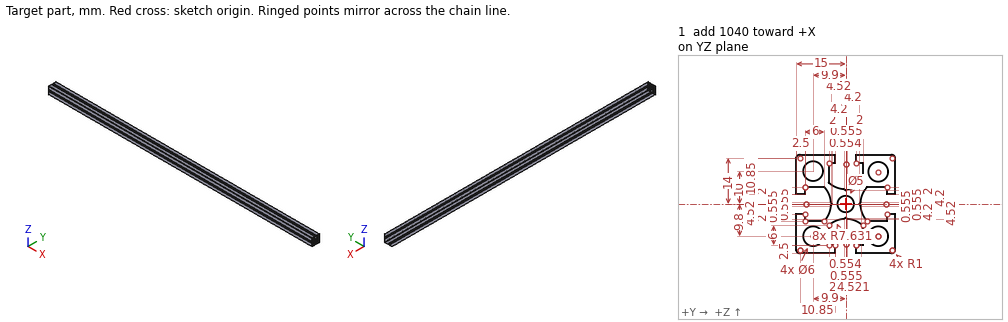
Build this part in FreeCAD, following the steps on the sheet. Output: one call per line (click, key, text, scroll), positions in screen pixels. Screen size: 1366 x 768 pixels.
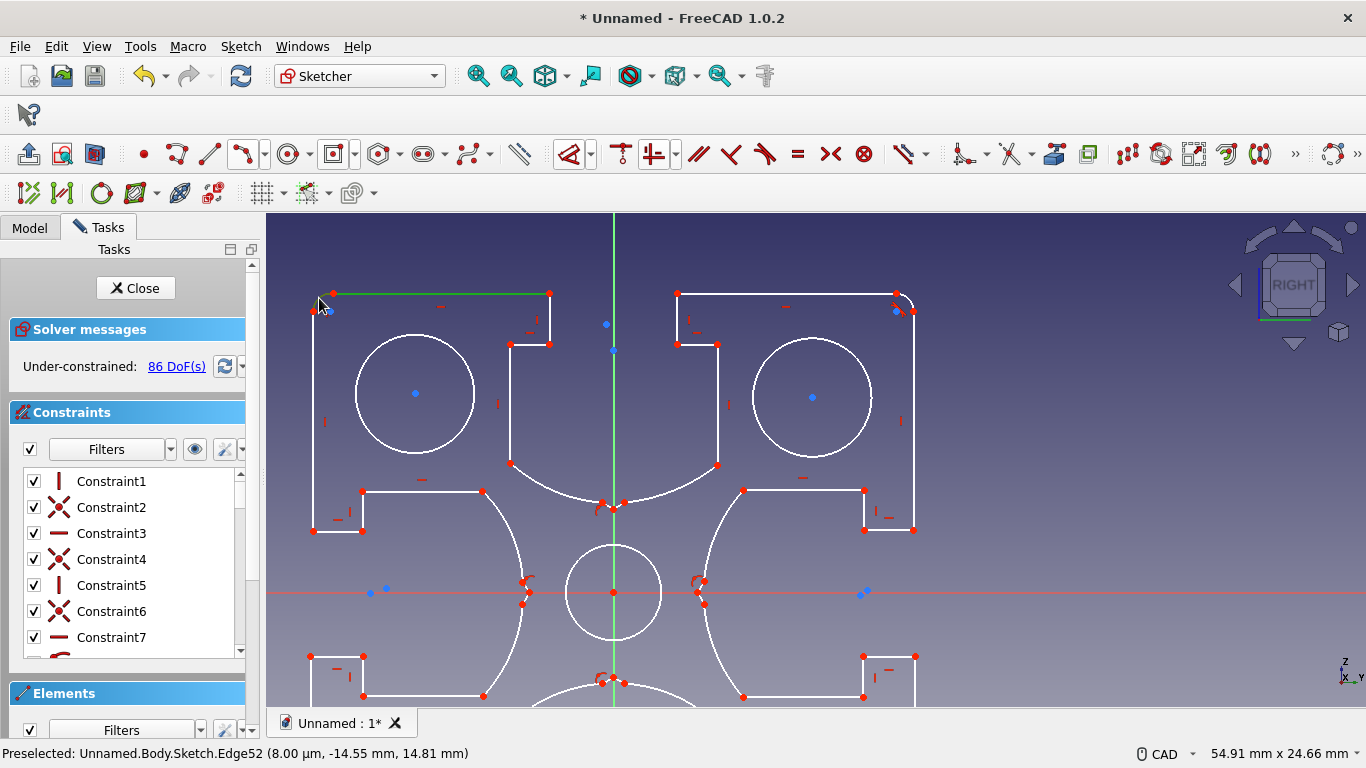
key(t)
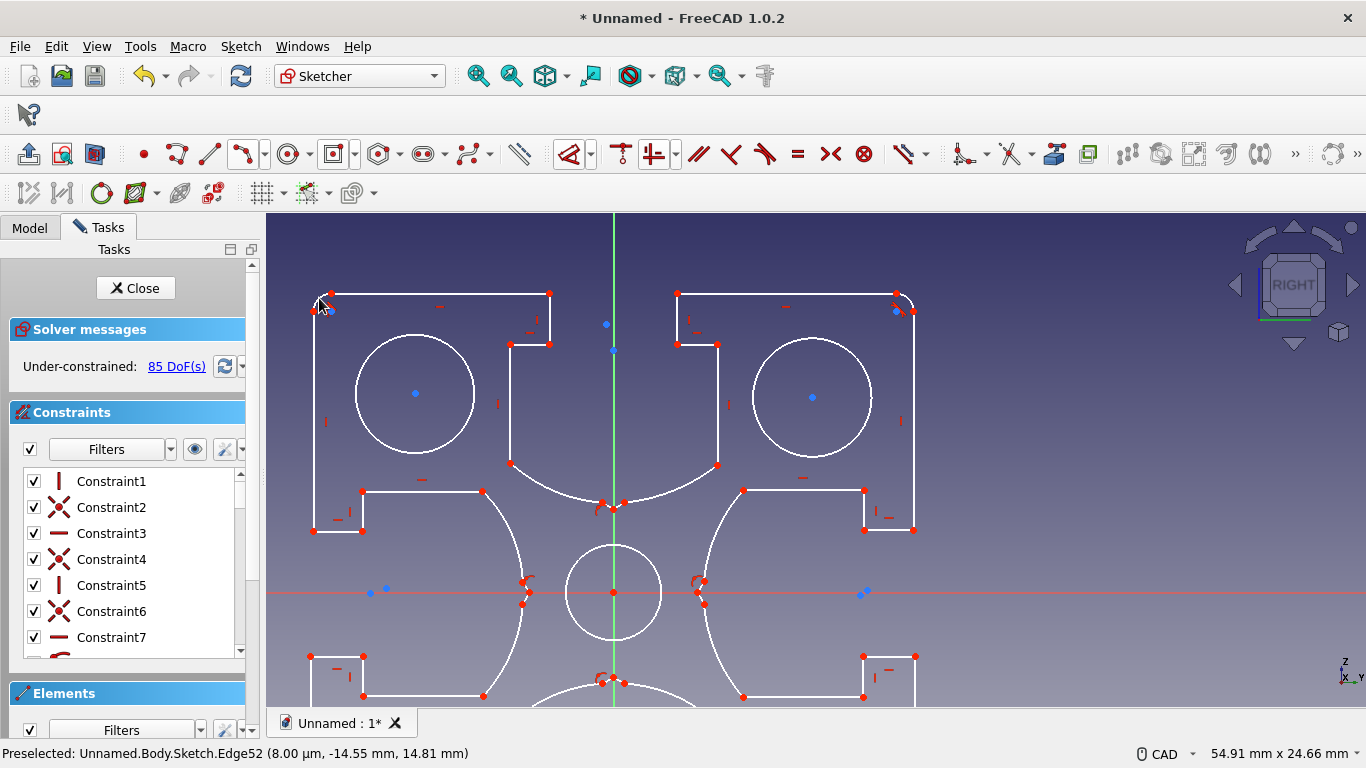
click(518, 552)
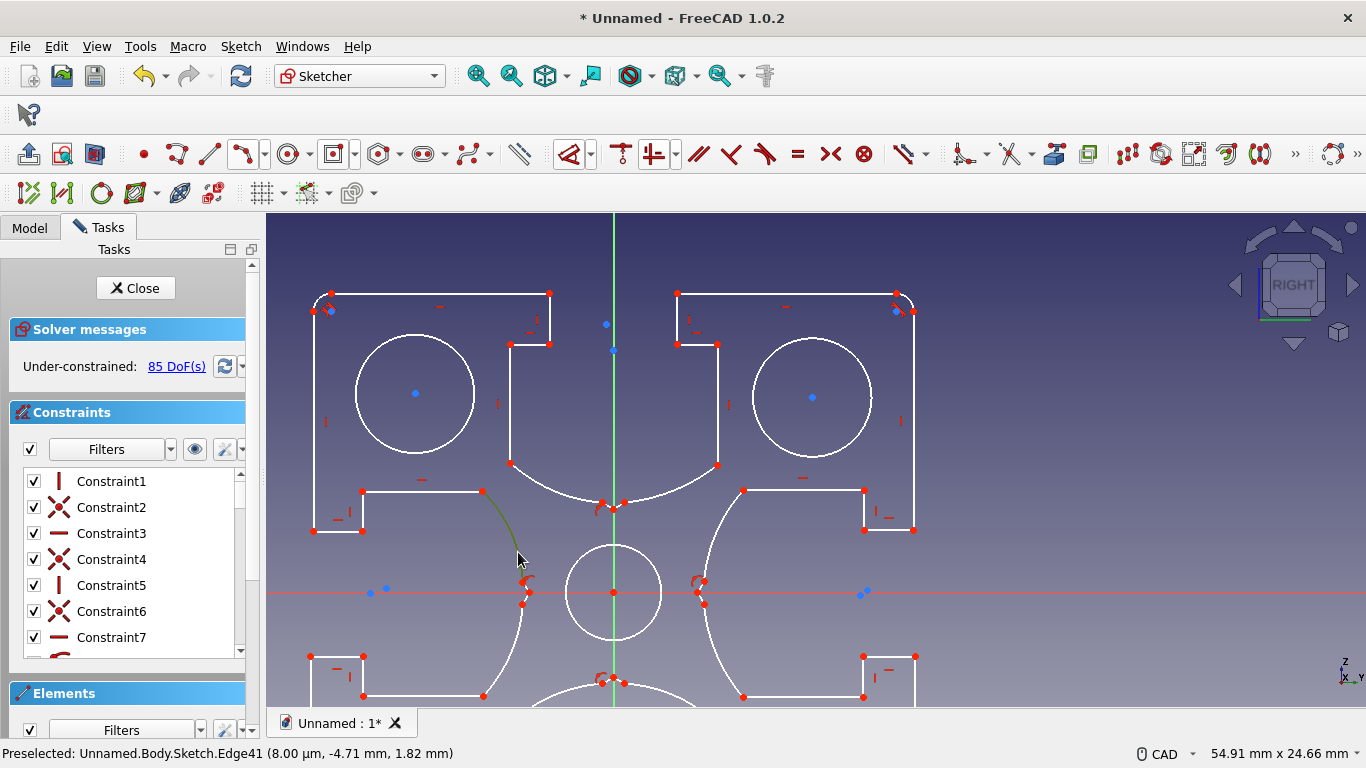
click(502, 672)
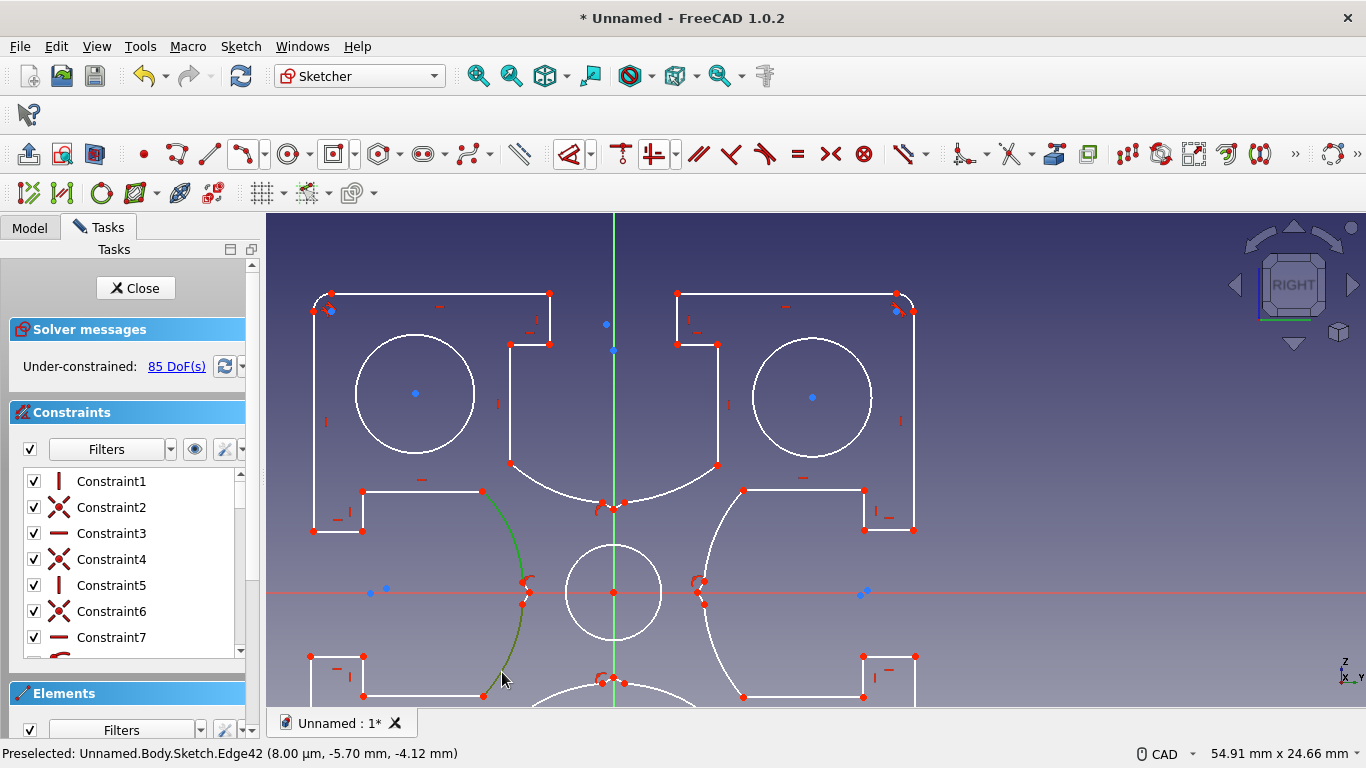
scroll(910, 299, down, 3)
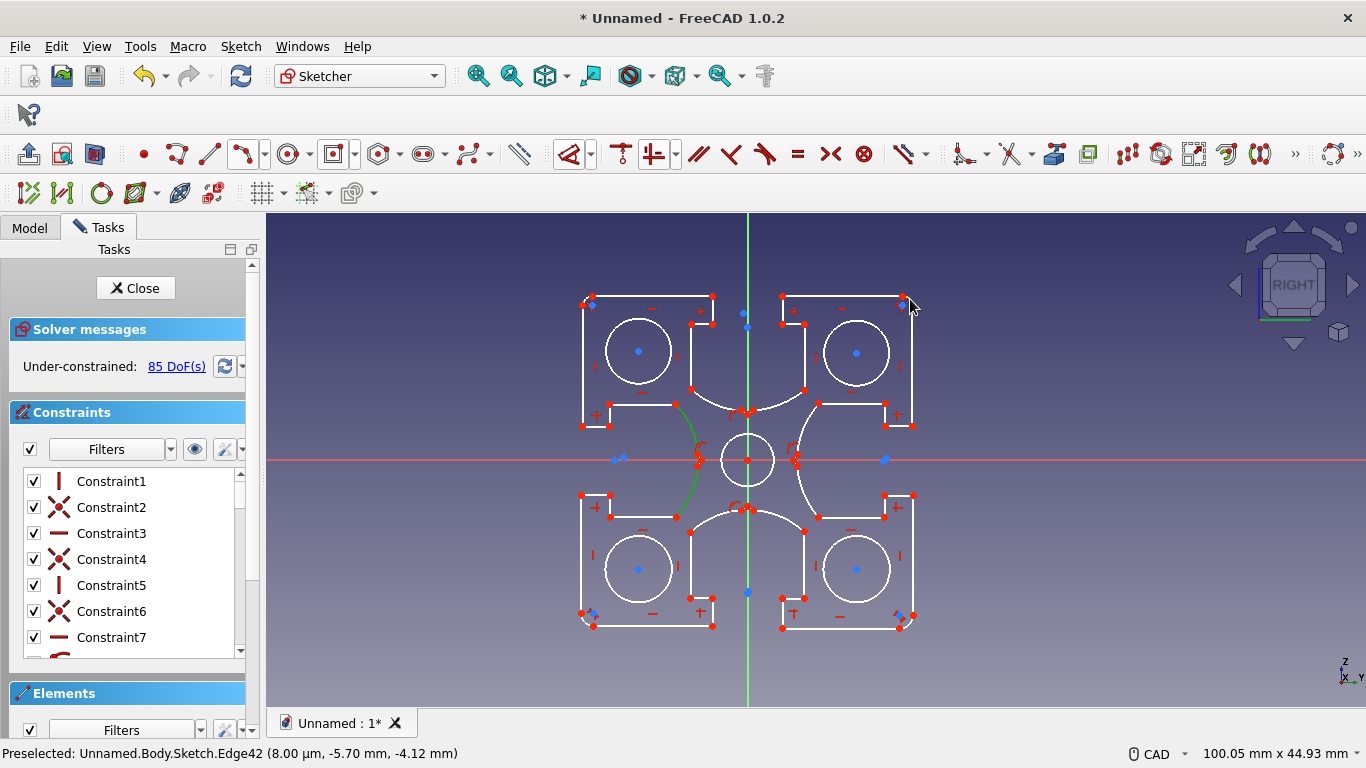
click(725, 513)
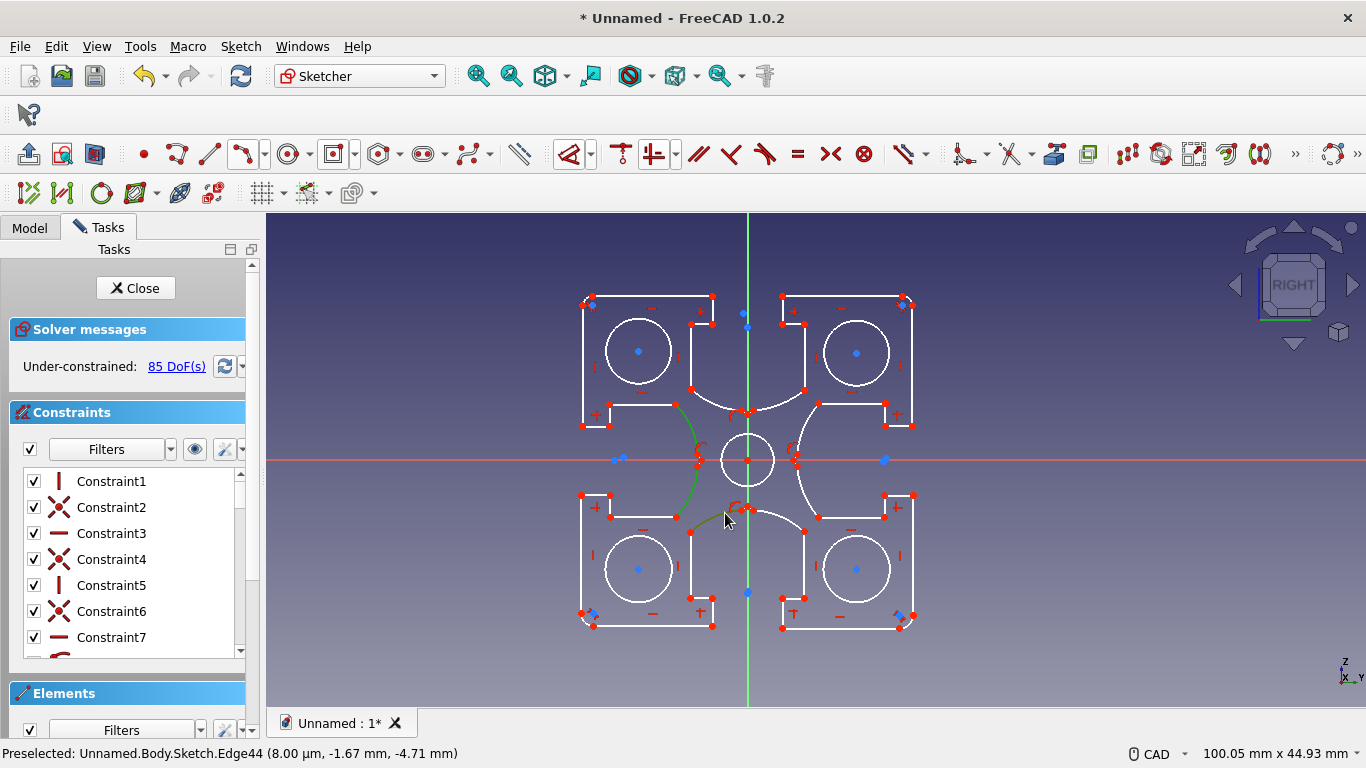
click(791, 522)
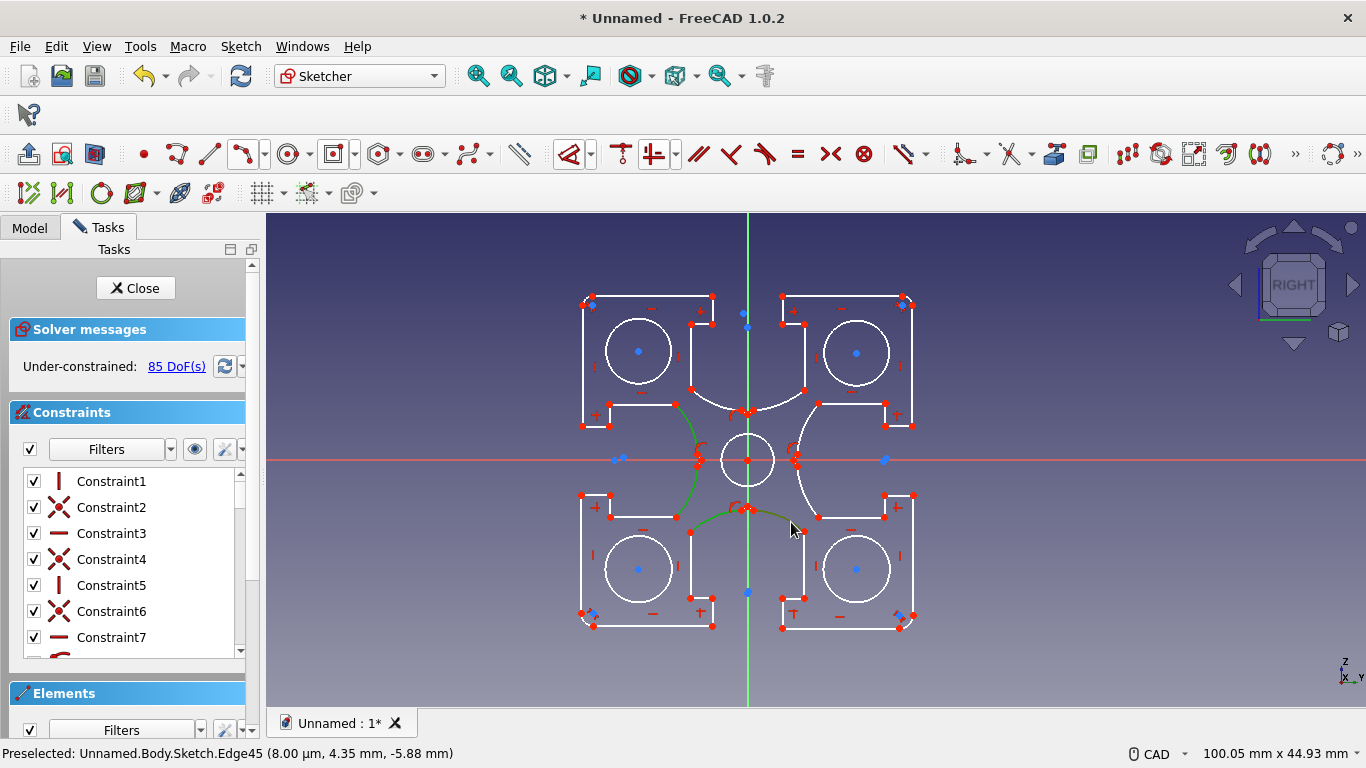
click(800, 483)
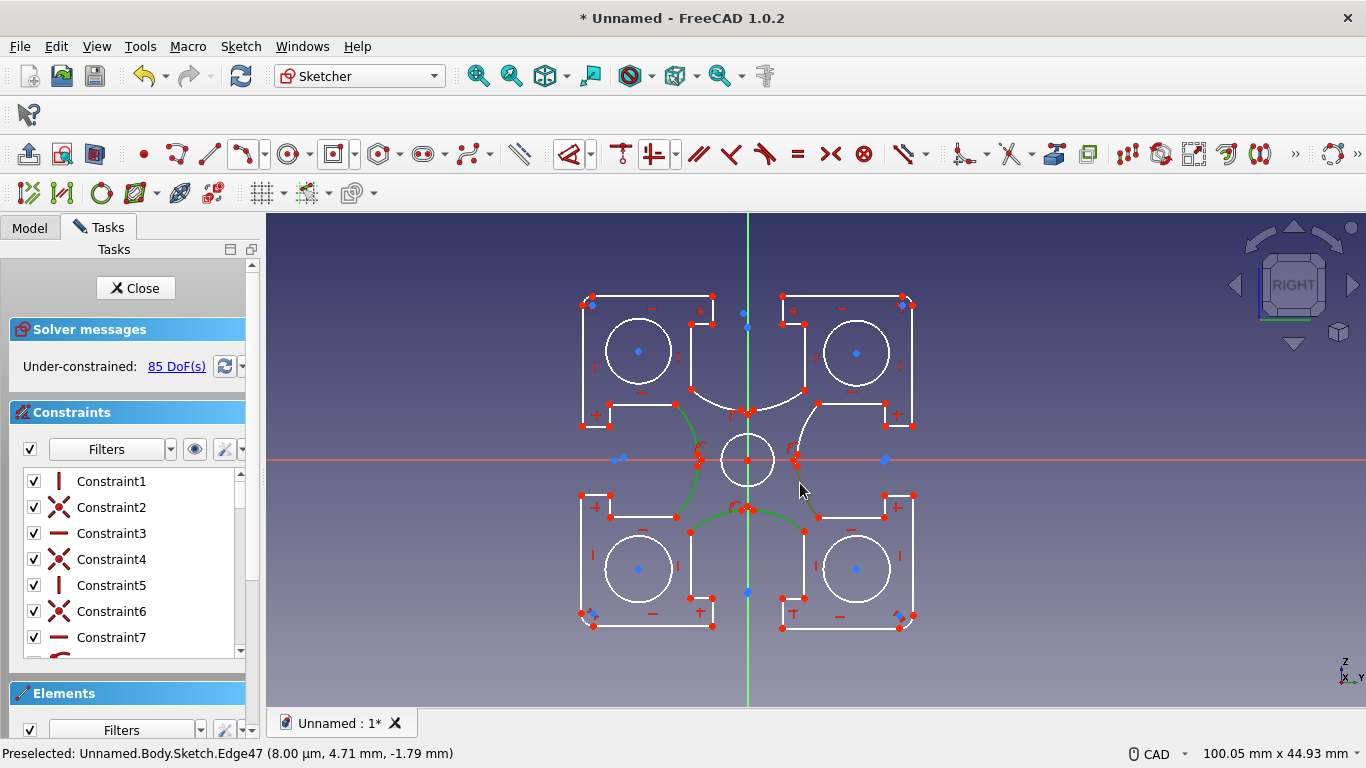
click(809, 417)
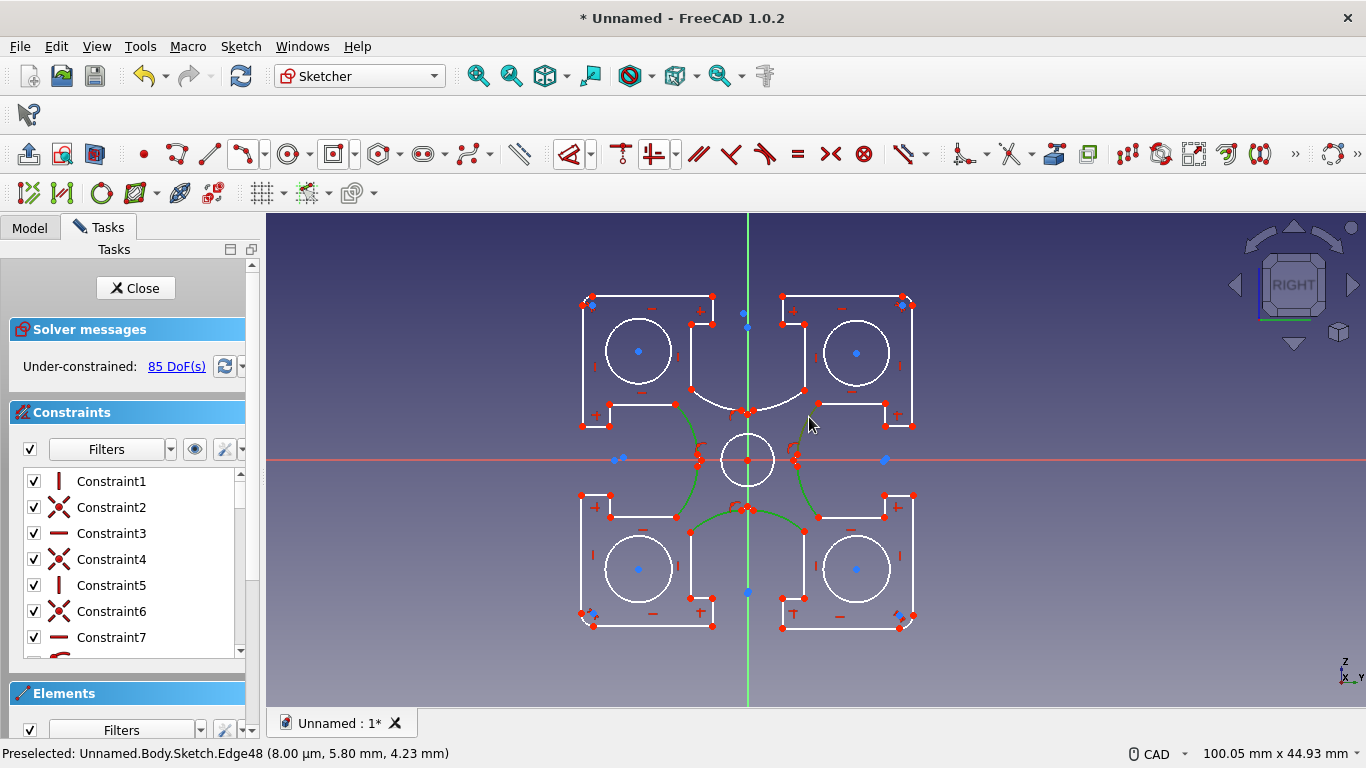
click(770, 408)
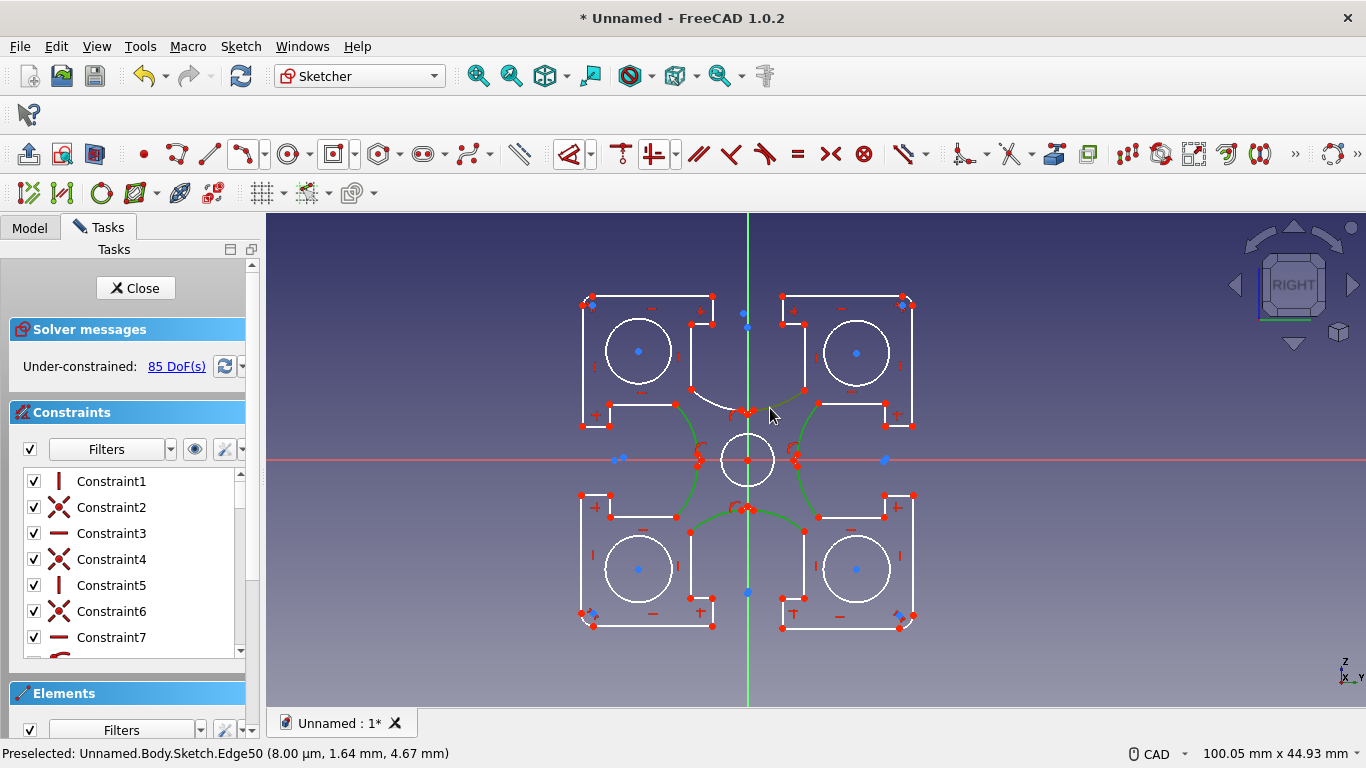
click(704, 399)